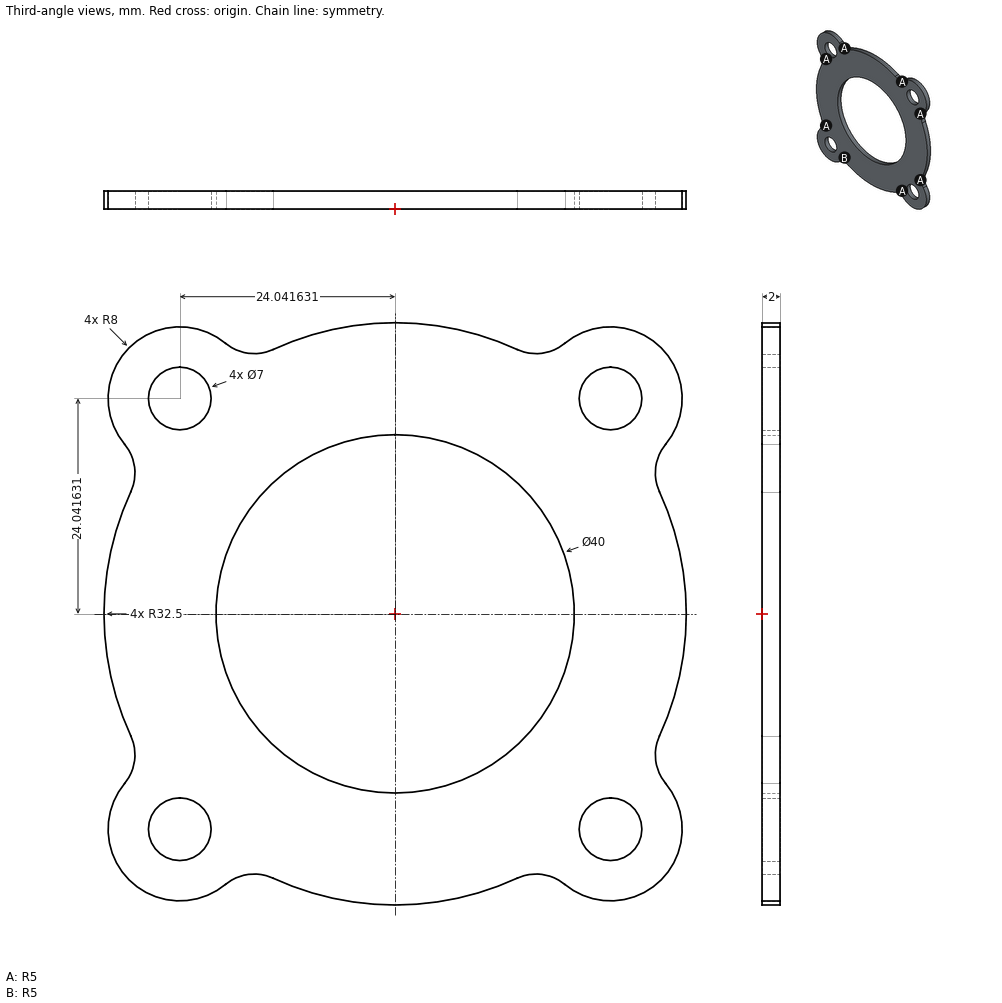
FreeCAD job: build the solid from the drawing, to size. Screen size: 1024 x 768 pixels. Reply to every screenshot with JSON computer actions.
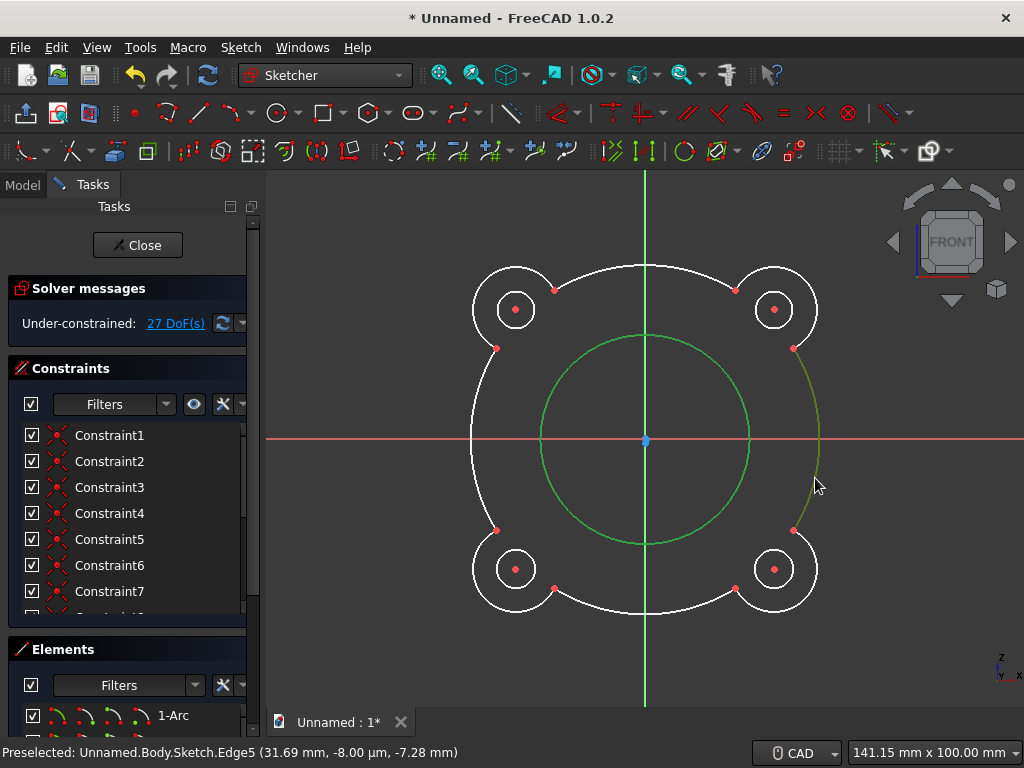
{"action": "left_click", "coordinate": [612, 114]}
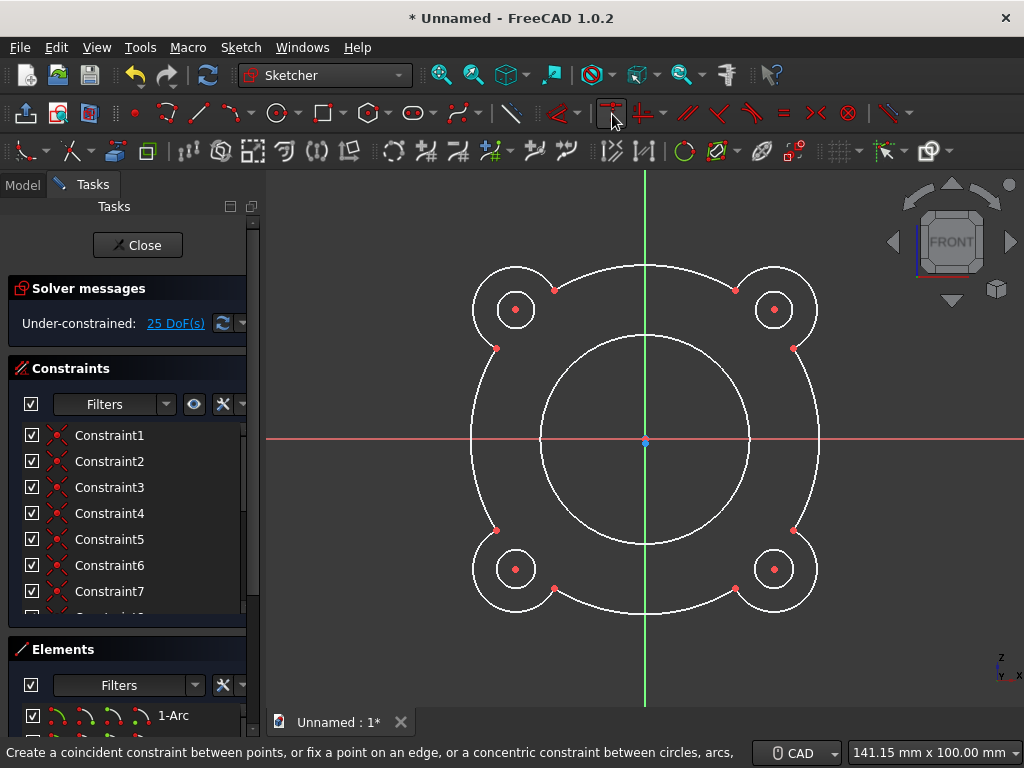
{"action": "left_click", "coordinate": [719, 365]}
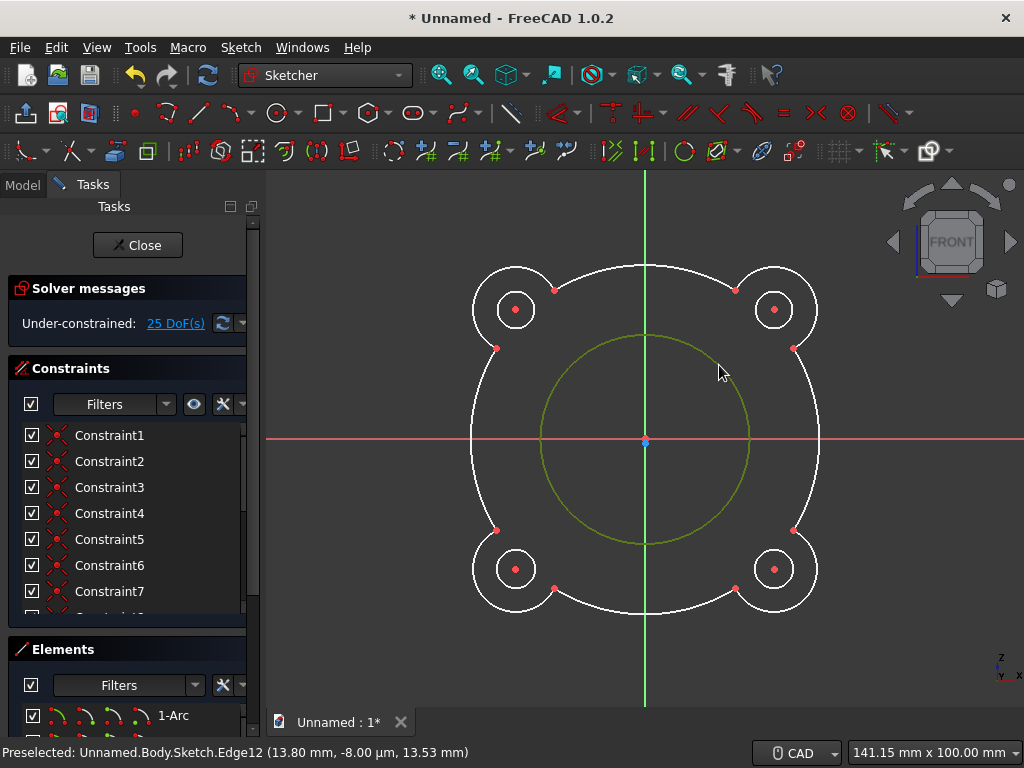
{"action": "left_click", "coordinate": [607, 610]}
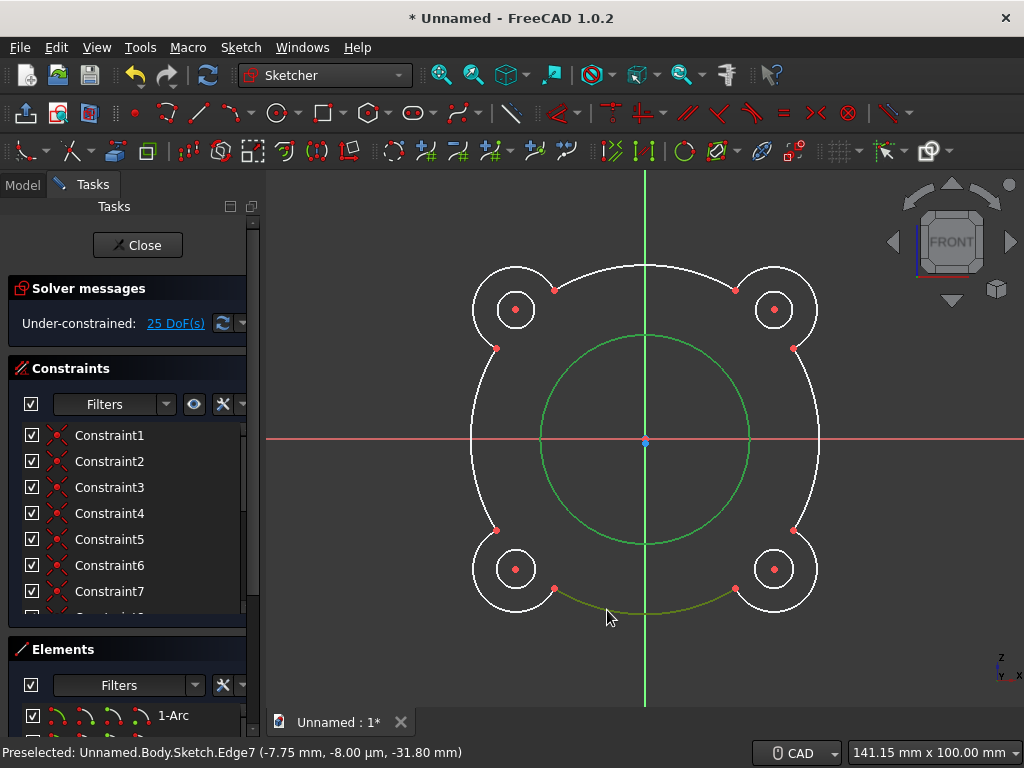
{"action": "left_click", "coordinate": [612, 114]}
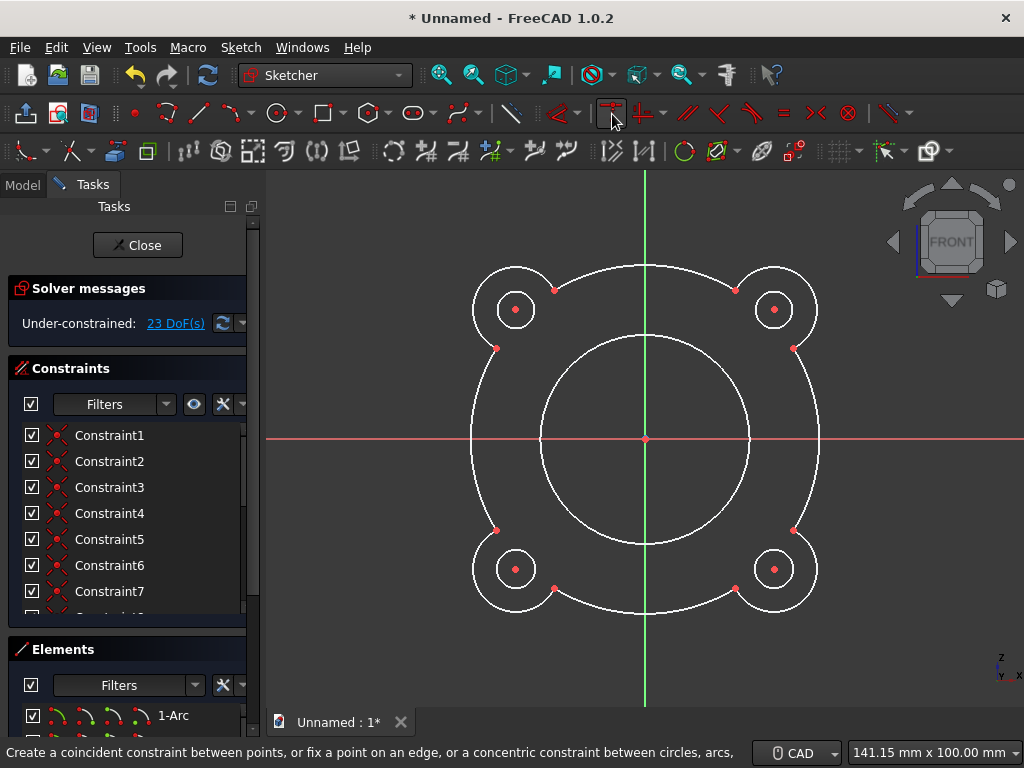
{"action": "scroll", "coordinate": [645, 439], "scroll_direction": "up", "scroll_amount": 4}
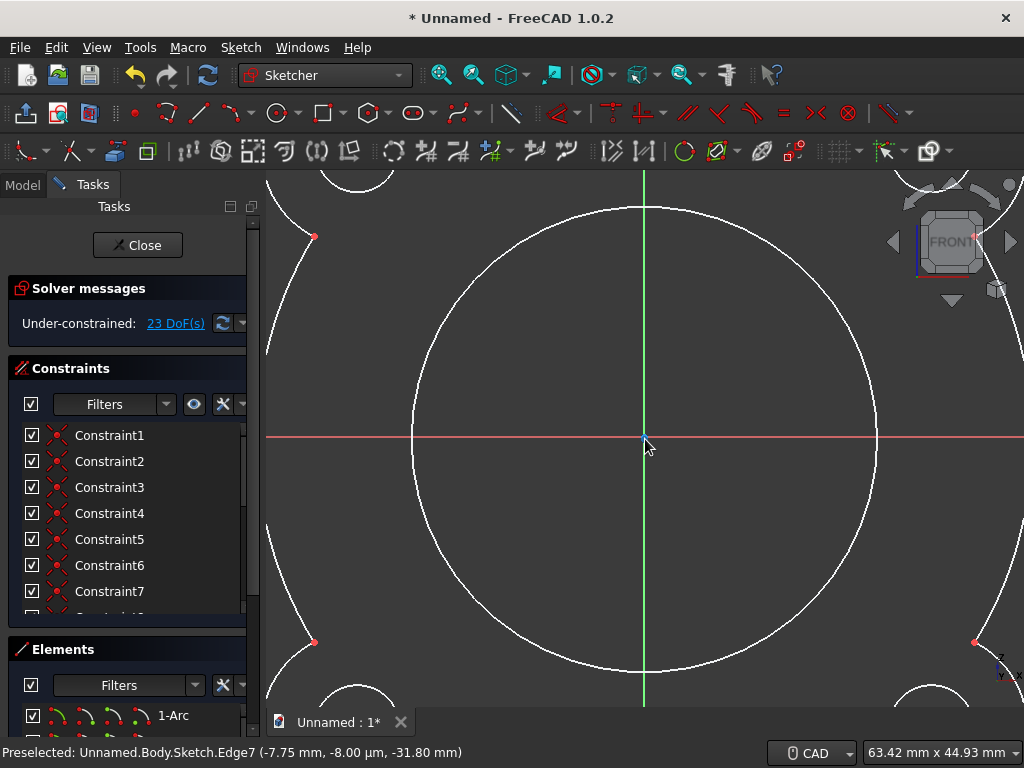
{"action": "left_click_drag", "start_coordinate": [634, 427], "coordinate": [654, 449]}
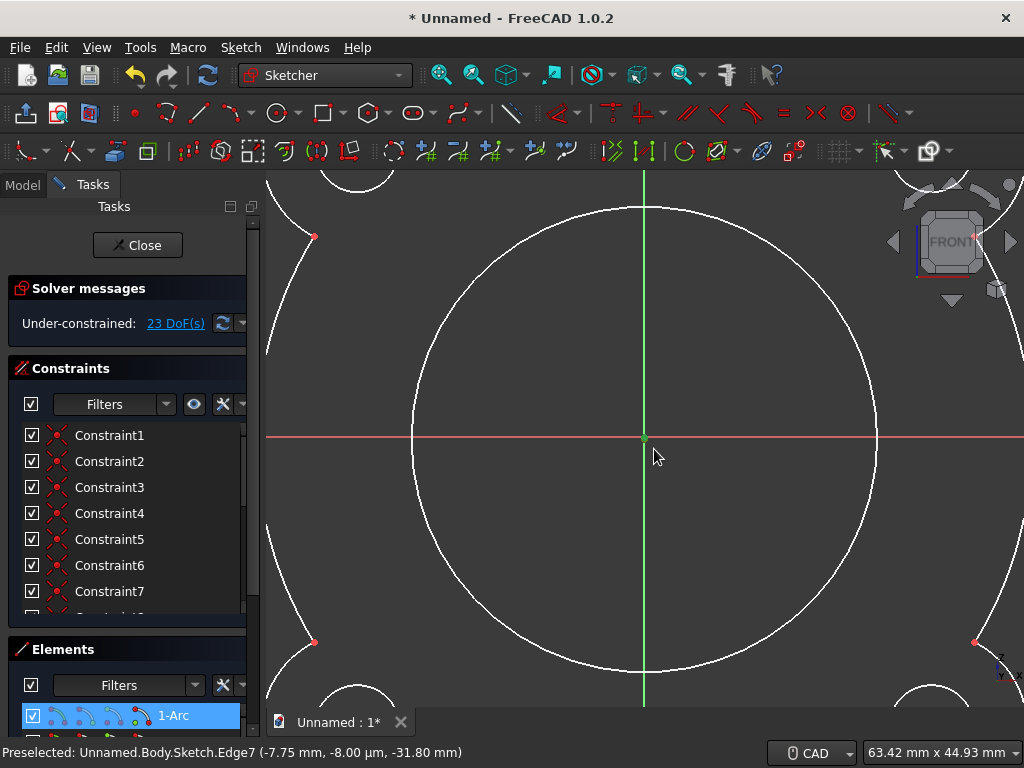
{"action": "left_click", "coordinate": [612, 114]}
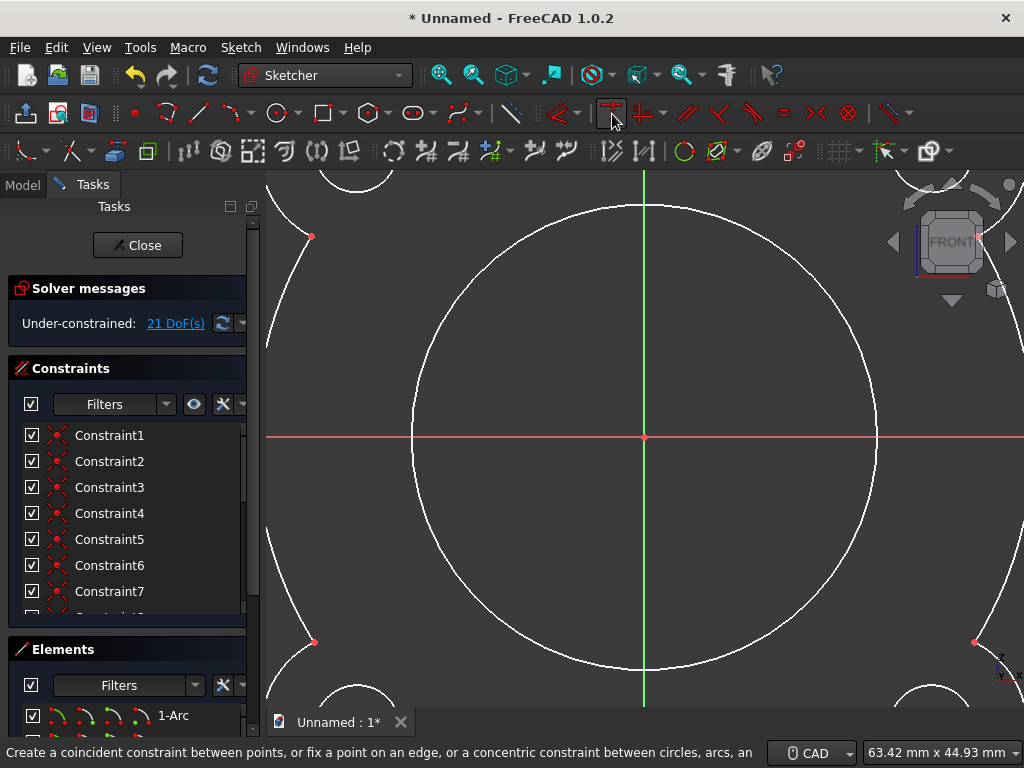
{"action": "scroll", "coordinate": [521, 440], "scroll_direction": "down", "scroll_amount": 4}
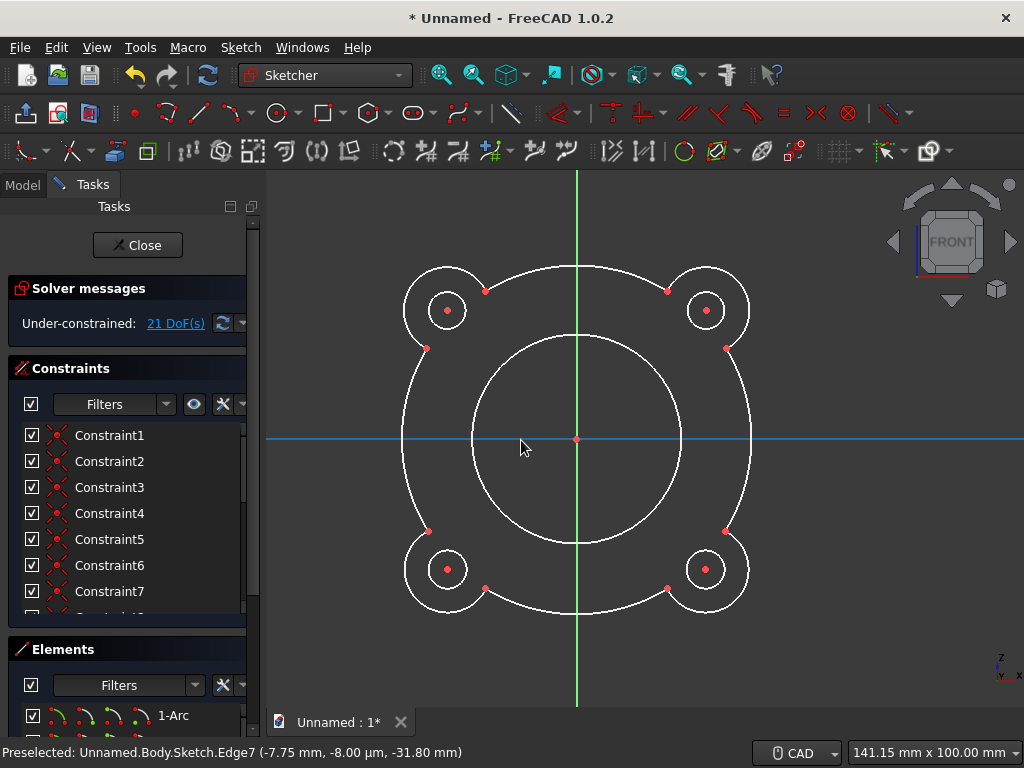
{"action": "left_click", "coordinate": [406, 402]}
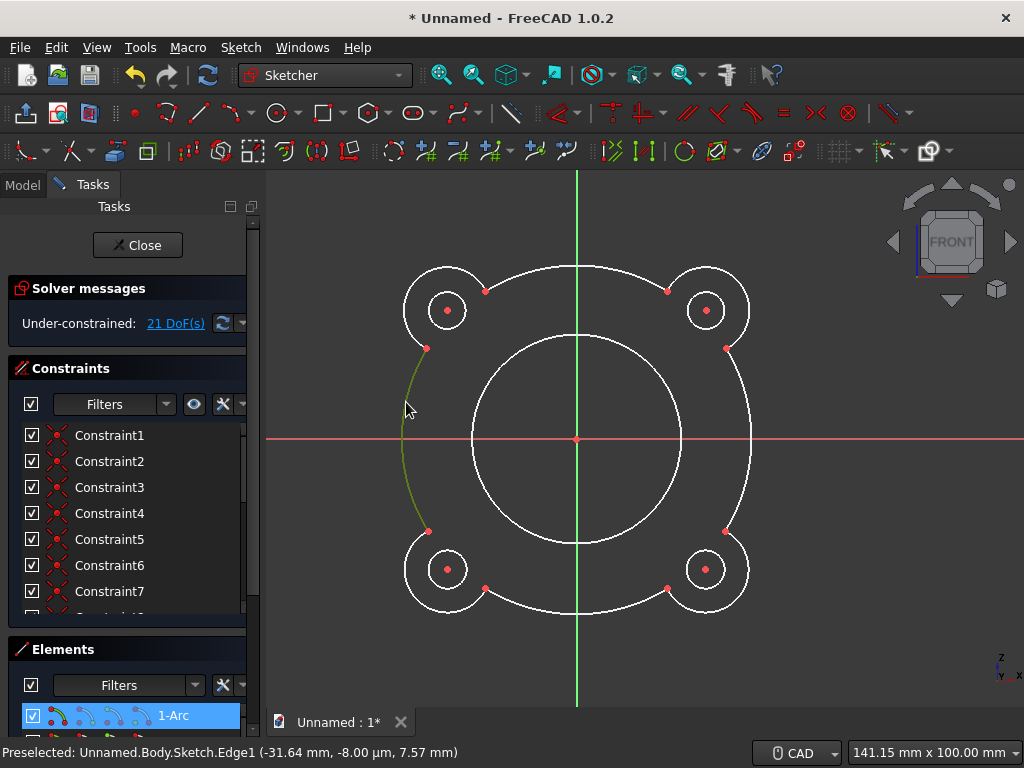
{"action": "left_click", "coordinate": [614, 270]}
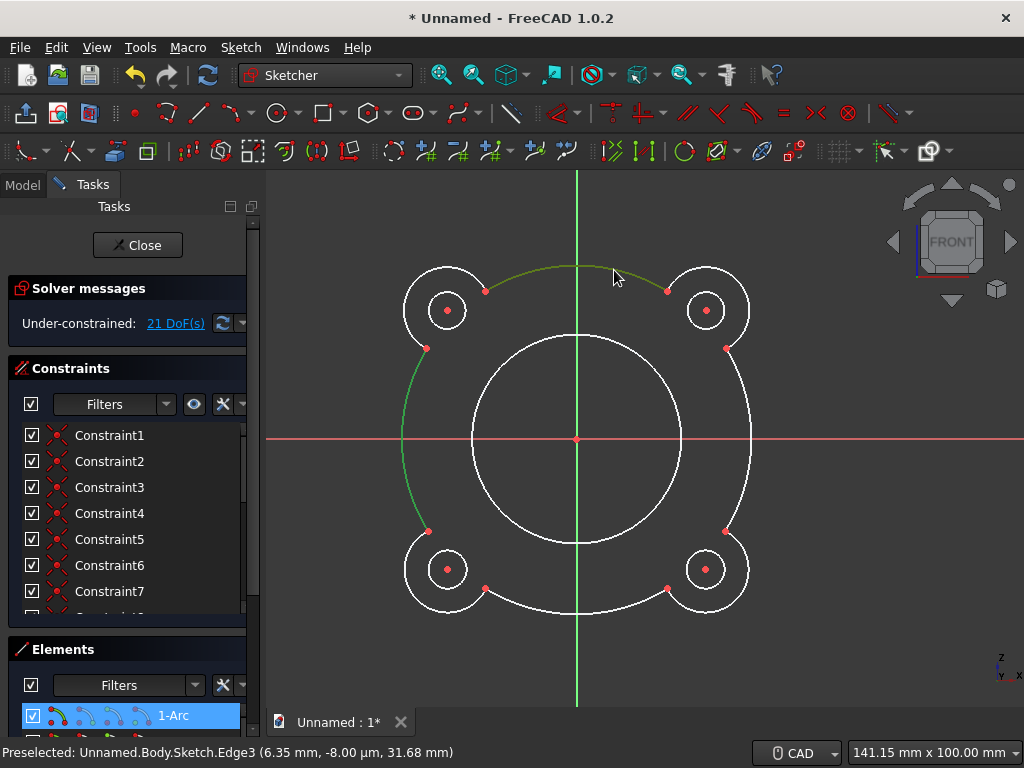
{"action": "left_click", "coordinate": [747, 478]}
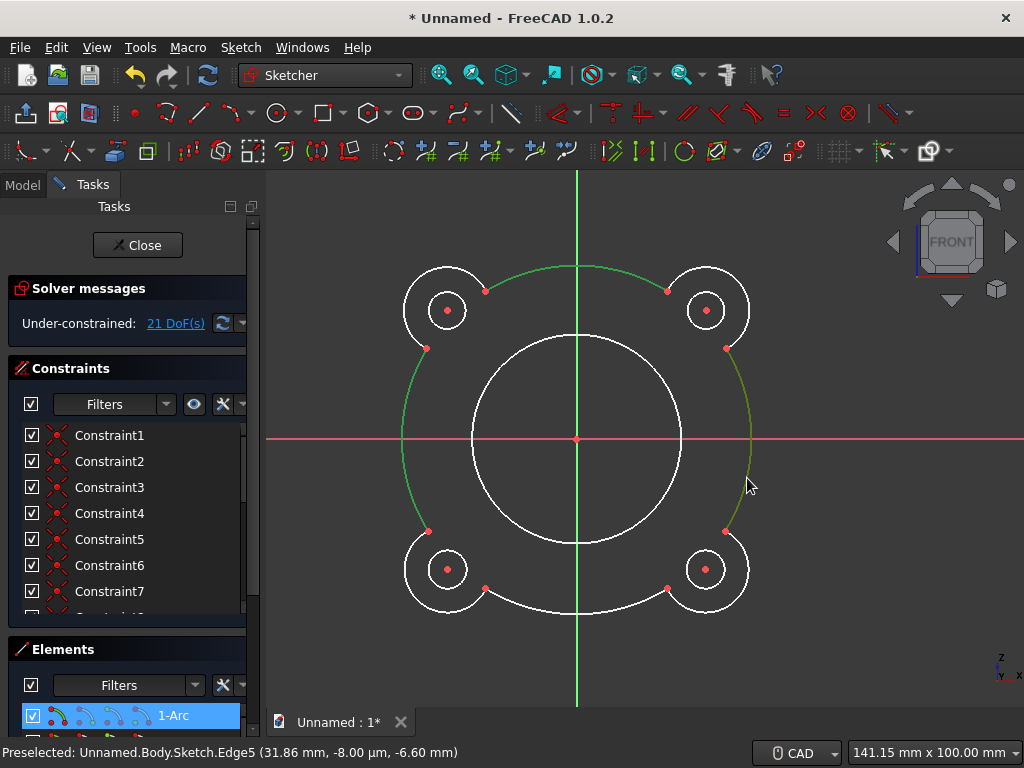
{"action": "left_click", "coordinate": [539, 610]}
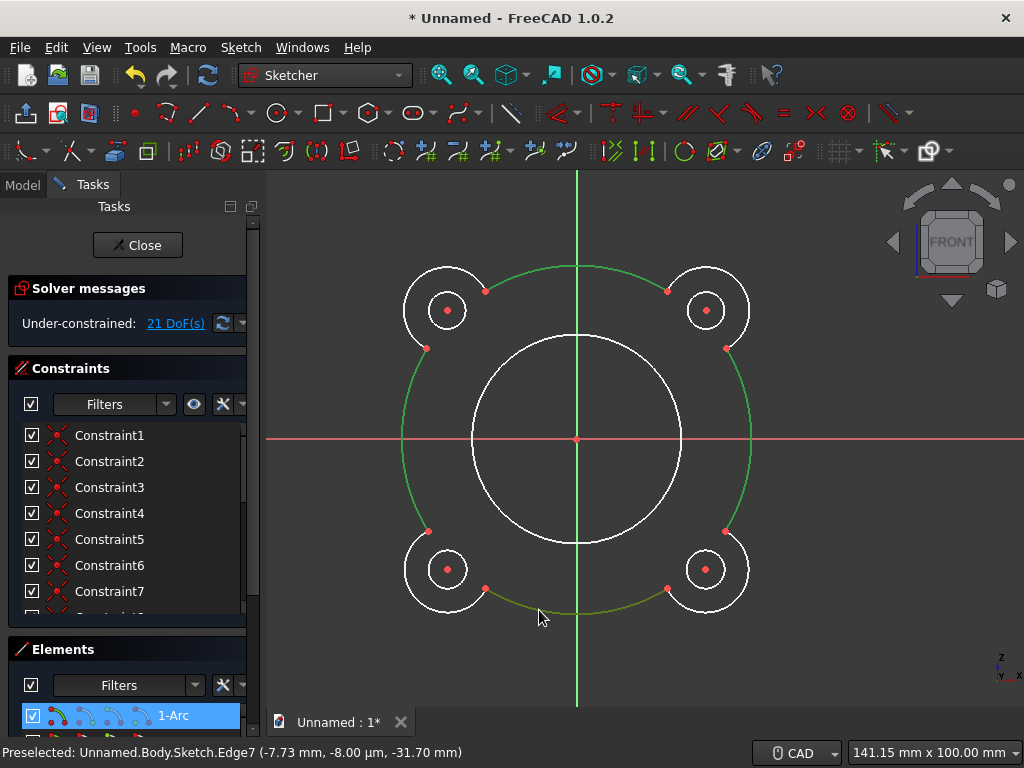
{"action": "key", "text": "e"}